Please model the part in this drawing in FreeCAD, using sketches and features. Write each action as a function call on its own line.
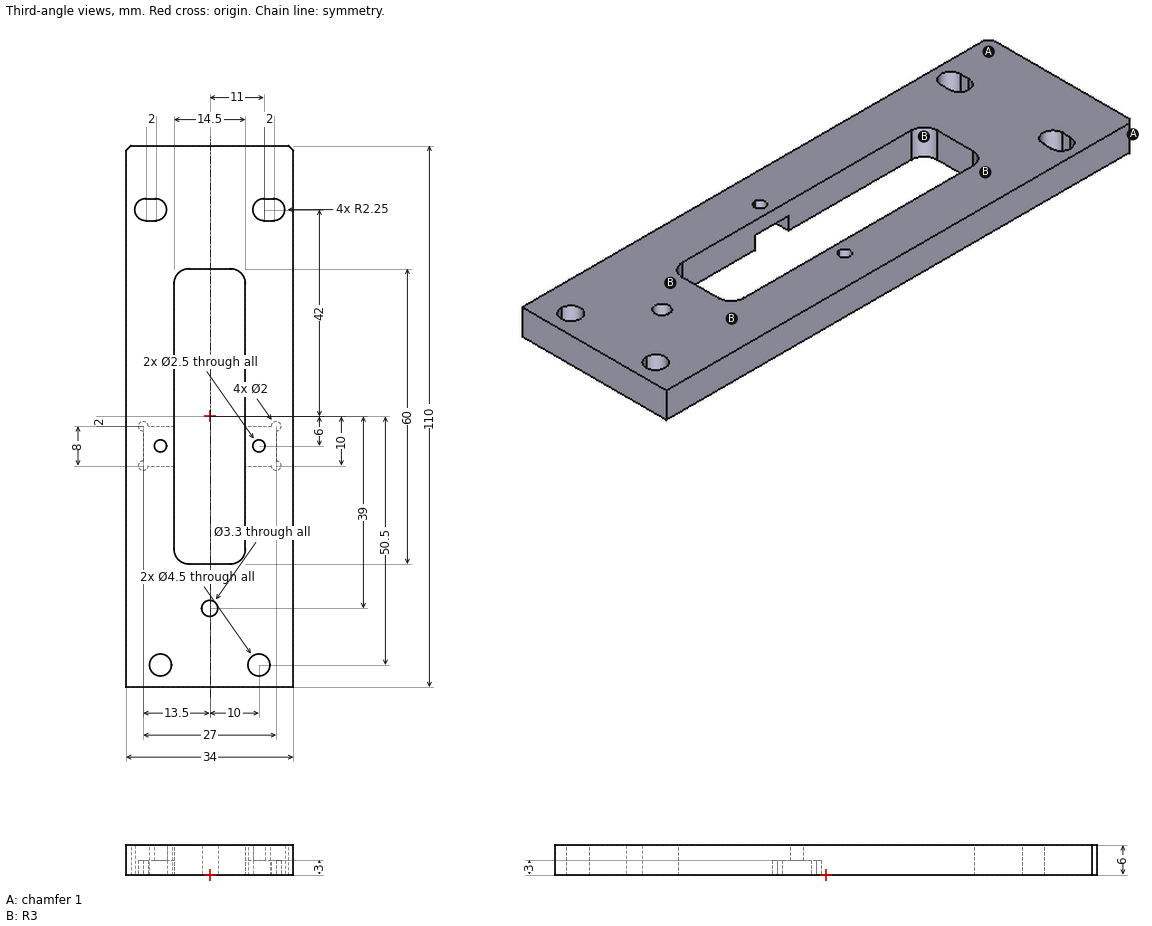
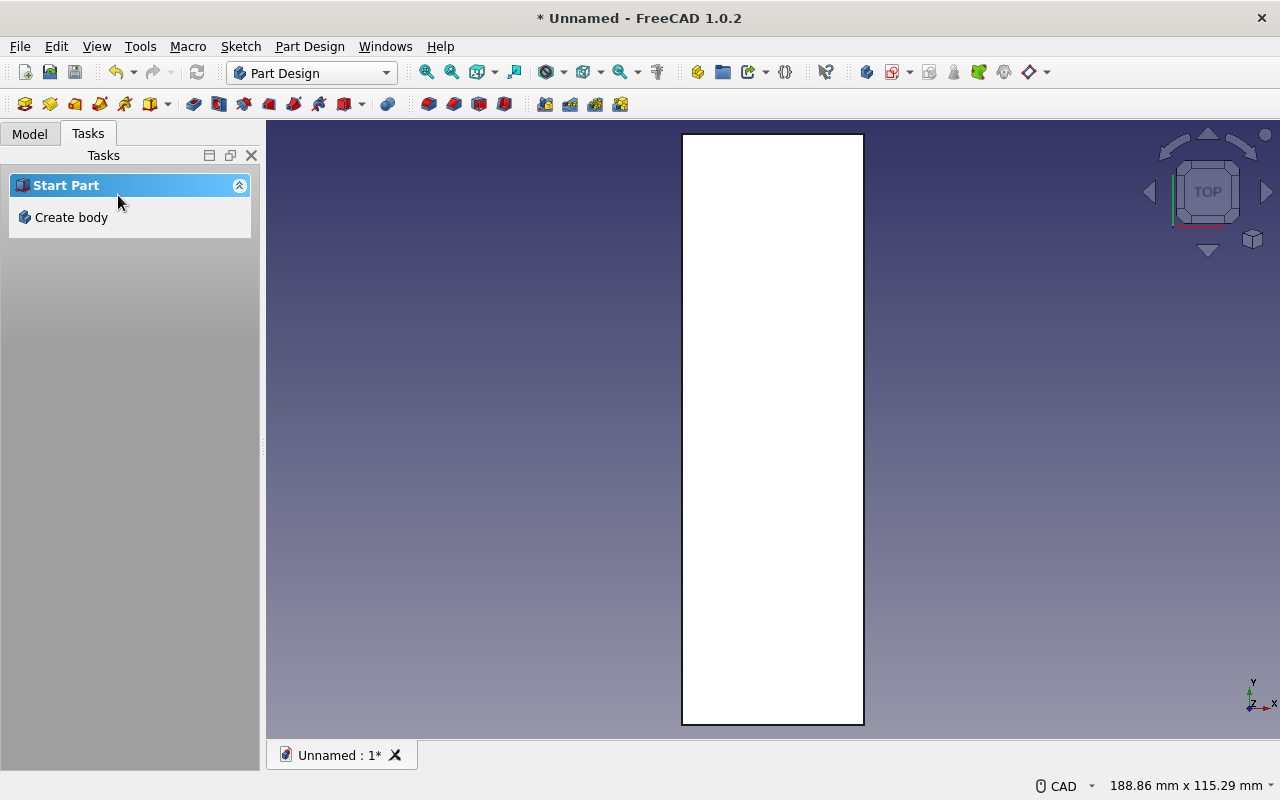
key(1)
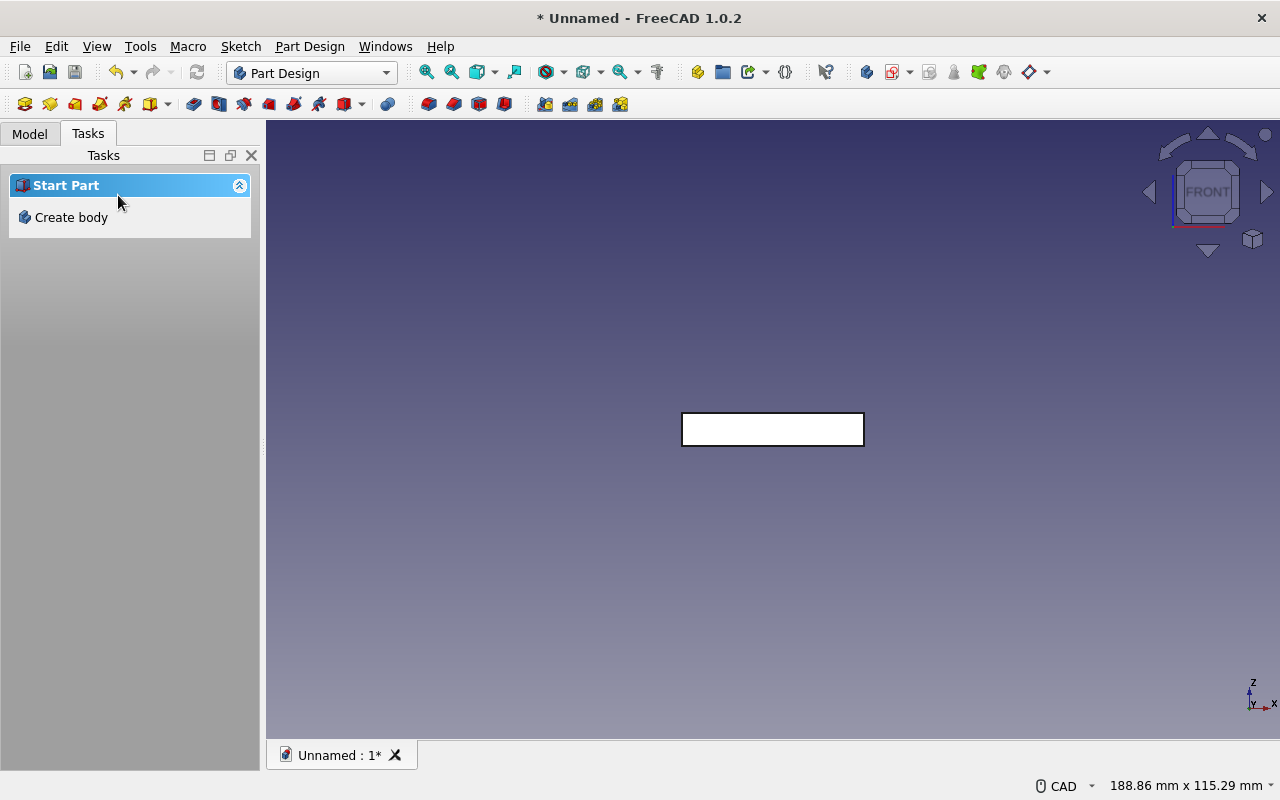
key(v)
key(f)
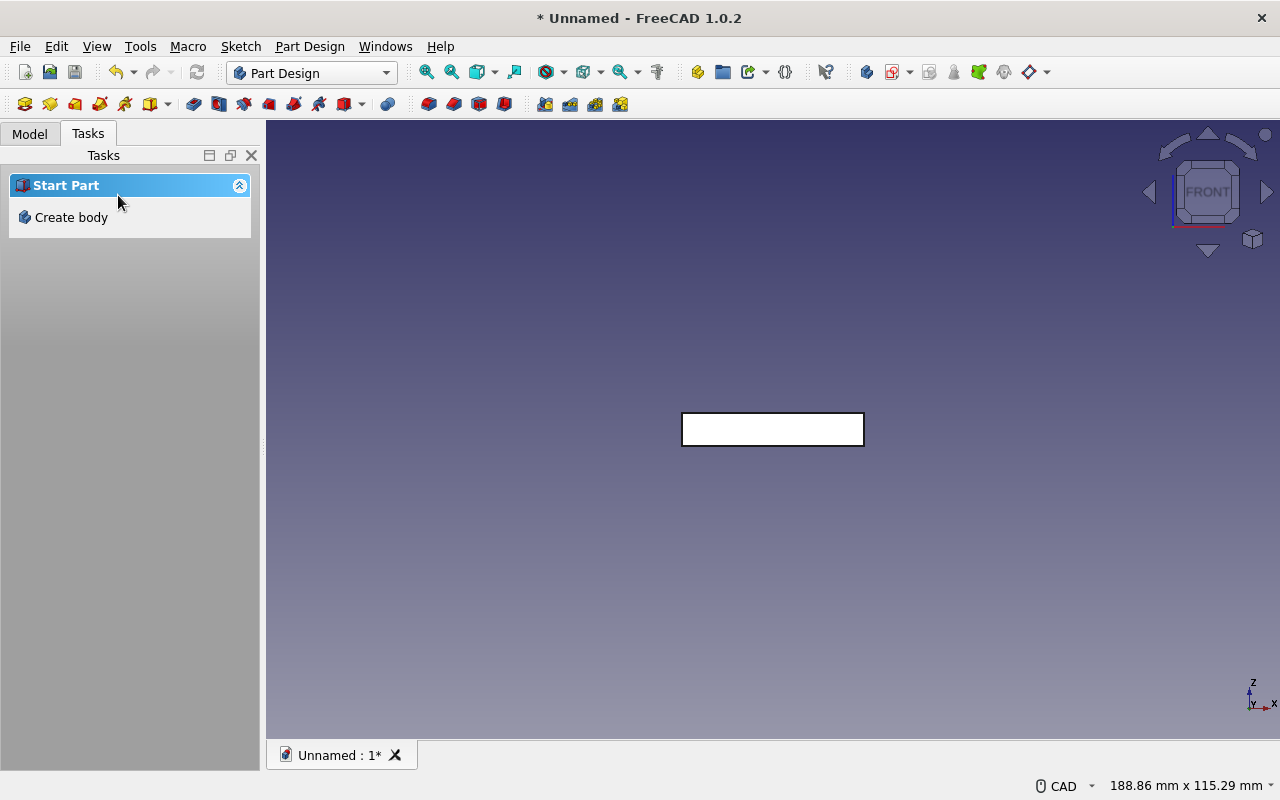
key(3)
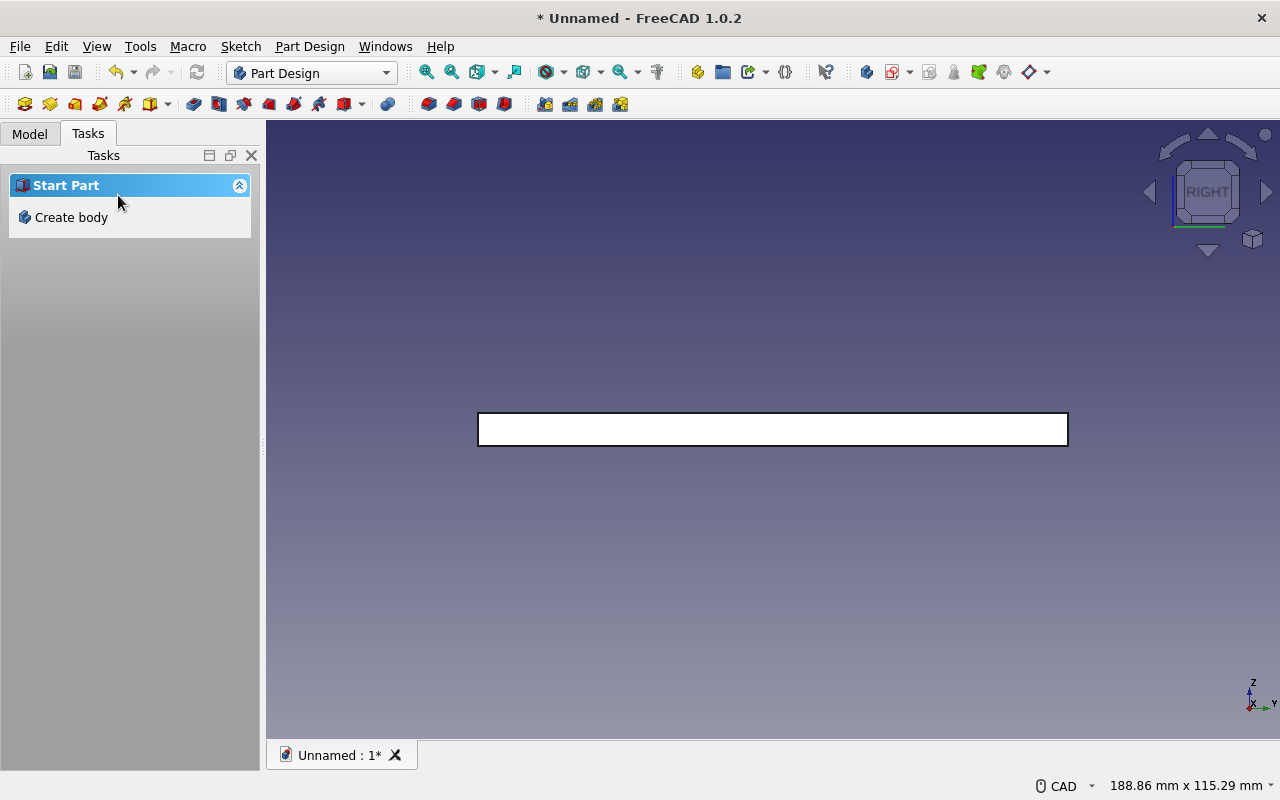
click(1068, 428)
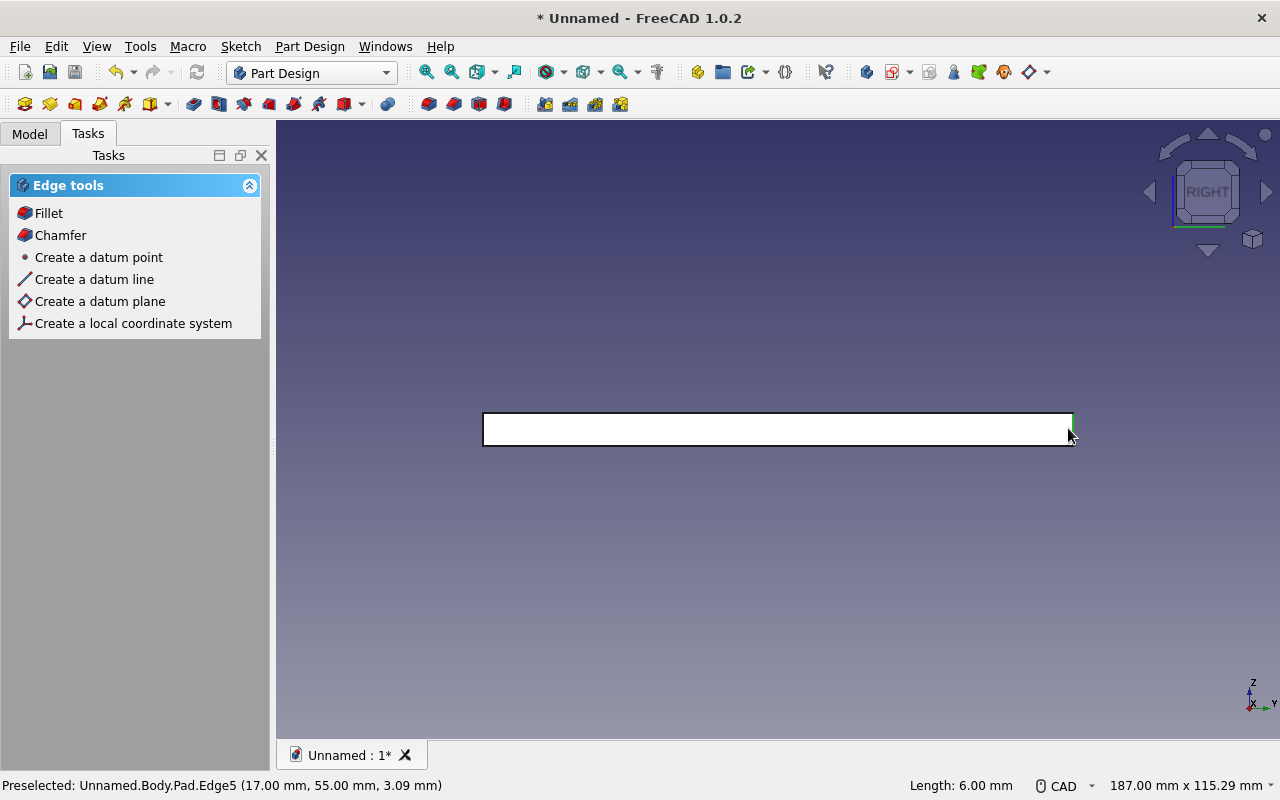
key(5)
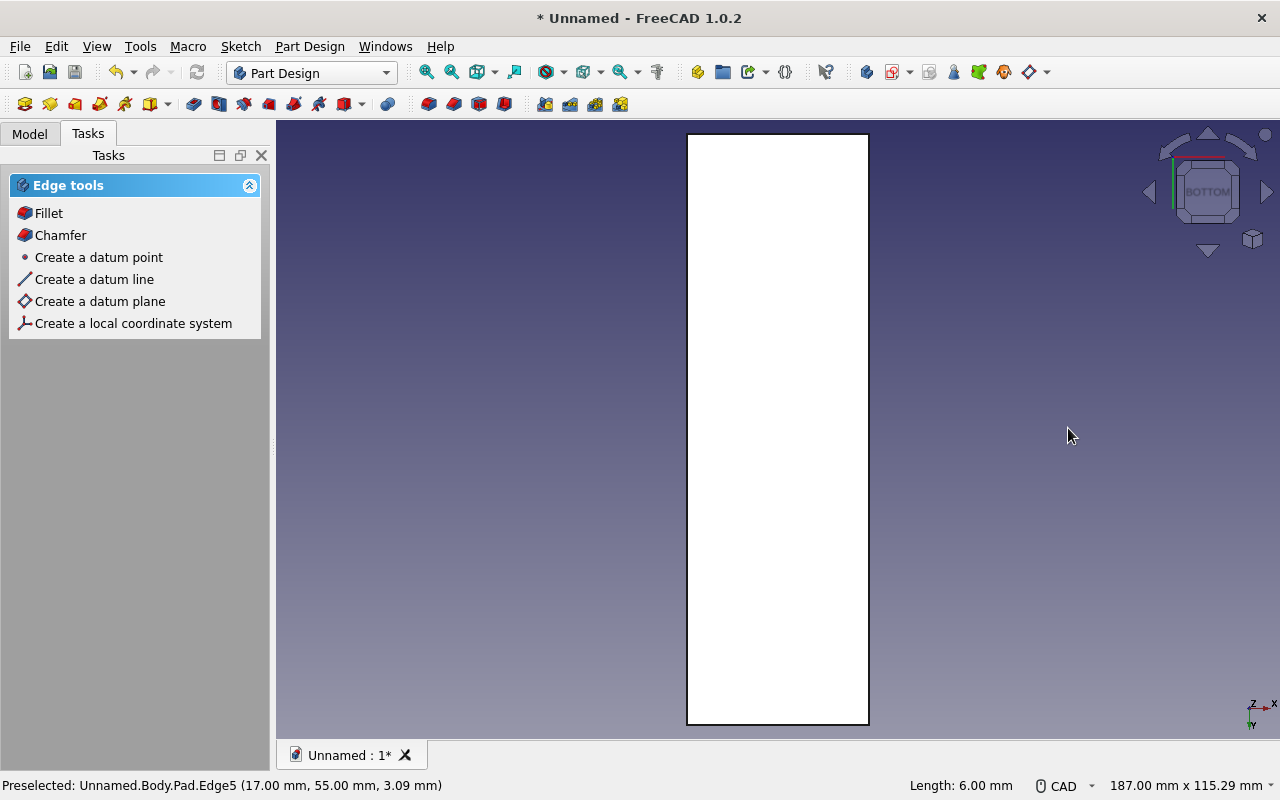
key(4)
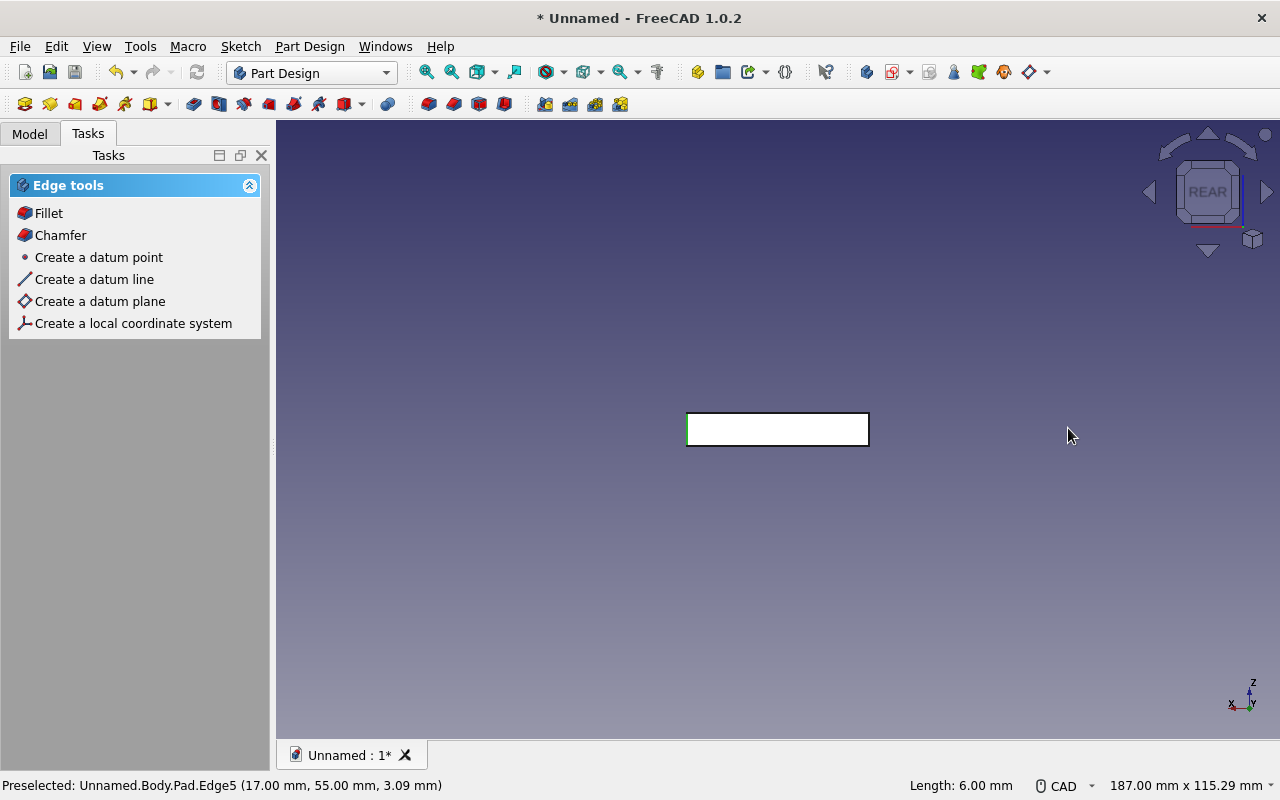
key(v)
key(f)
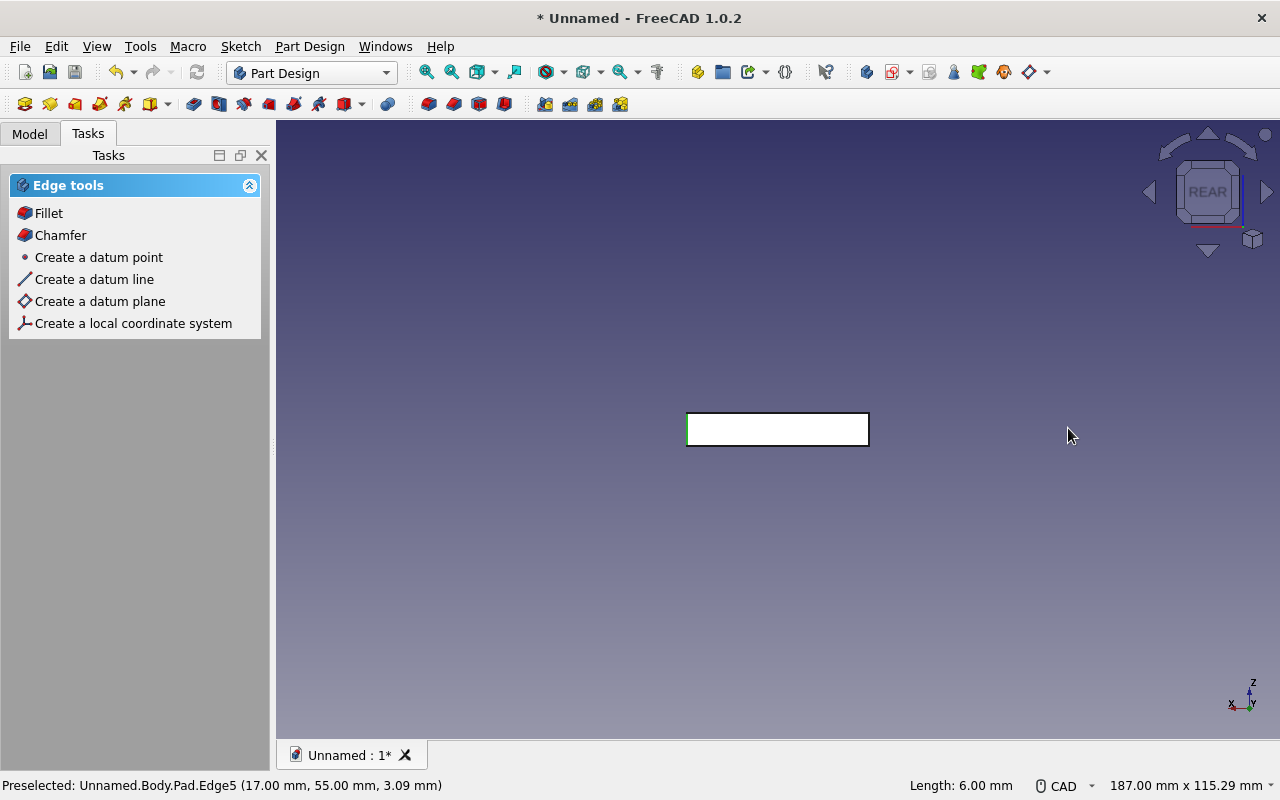
click(869, 429, ctrl)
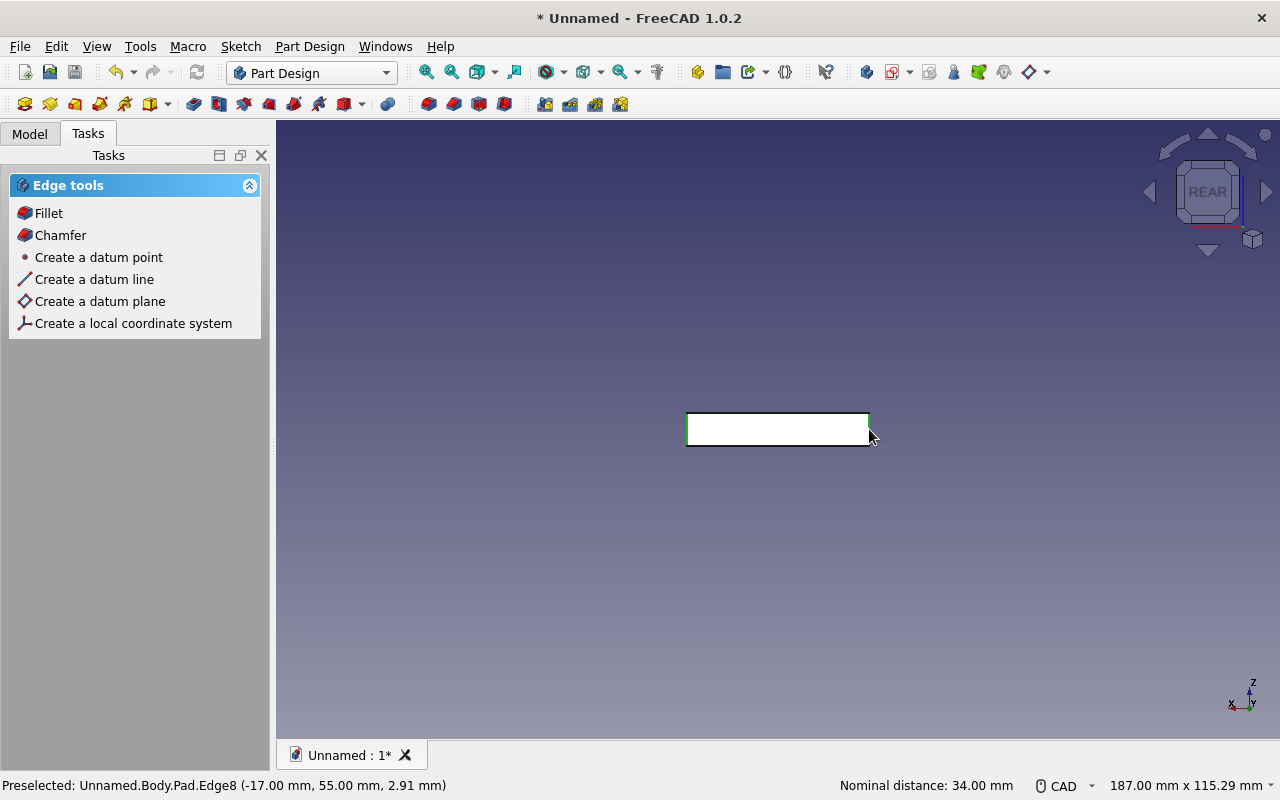
click(454, 104)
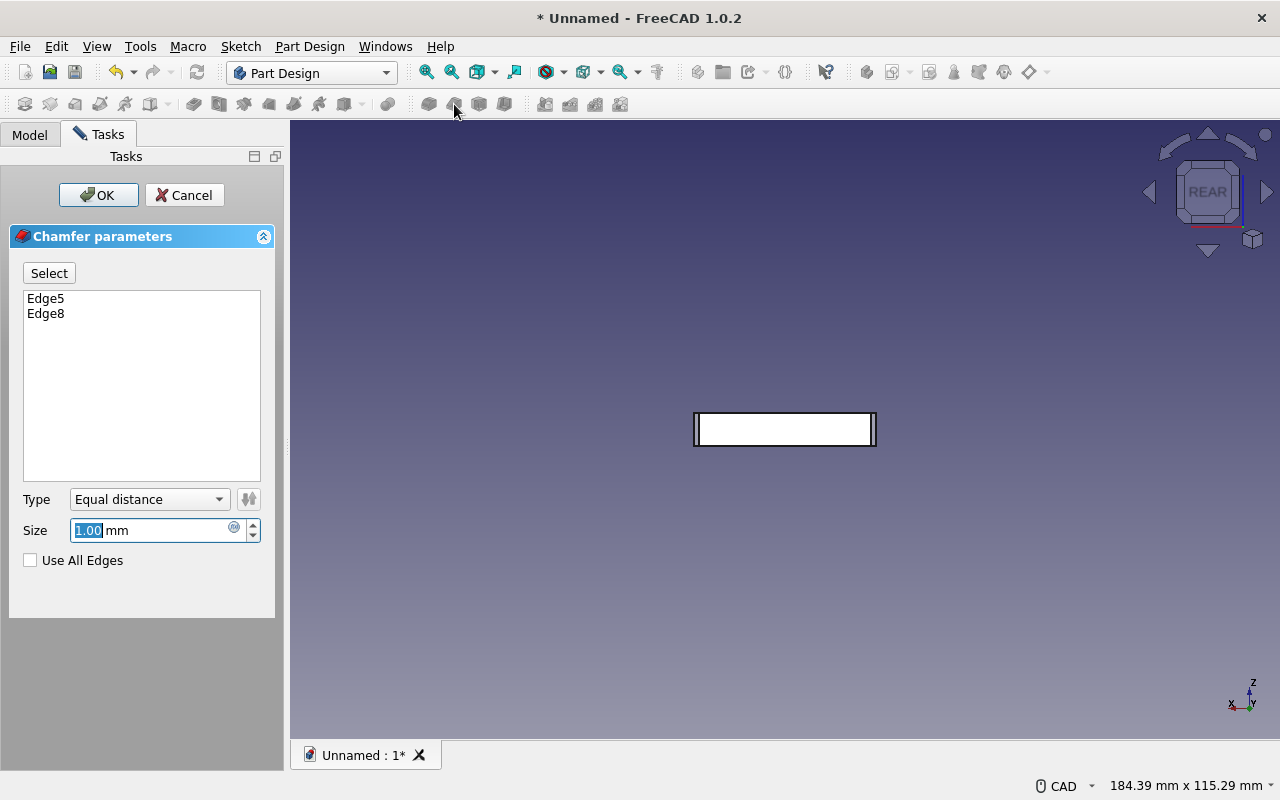
text(1)
key(Tab)